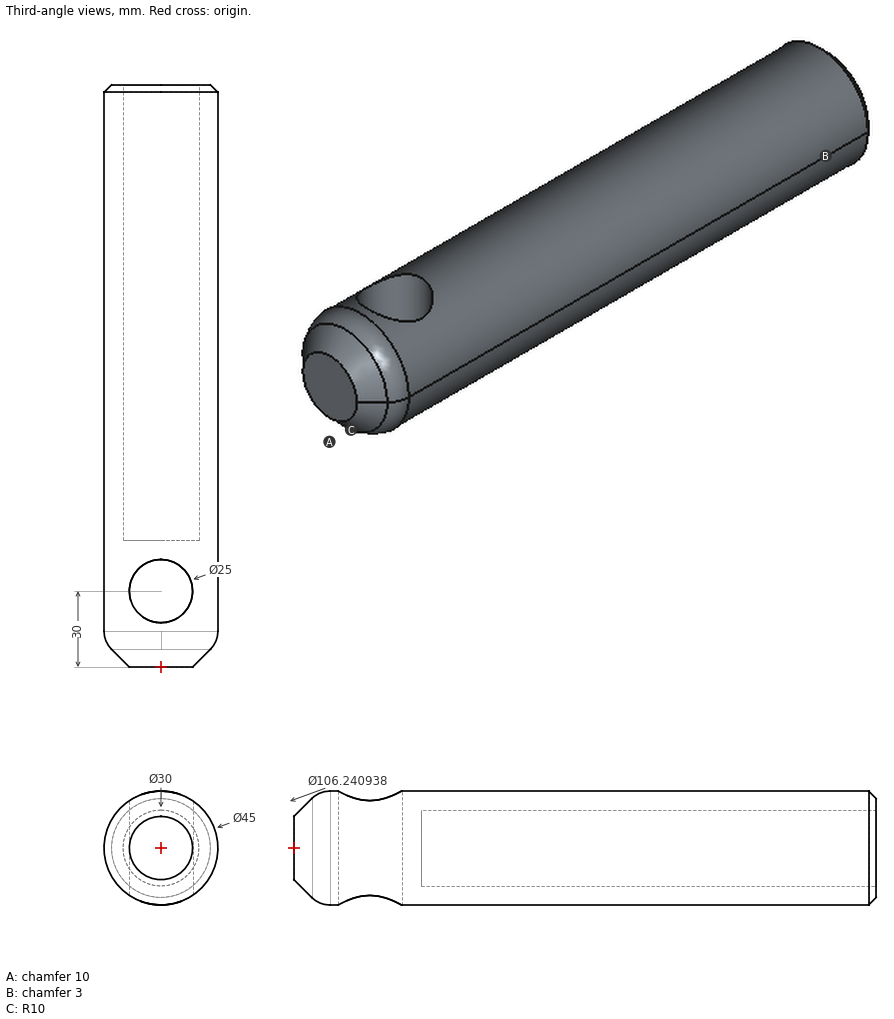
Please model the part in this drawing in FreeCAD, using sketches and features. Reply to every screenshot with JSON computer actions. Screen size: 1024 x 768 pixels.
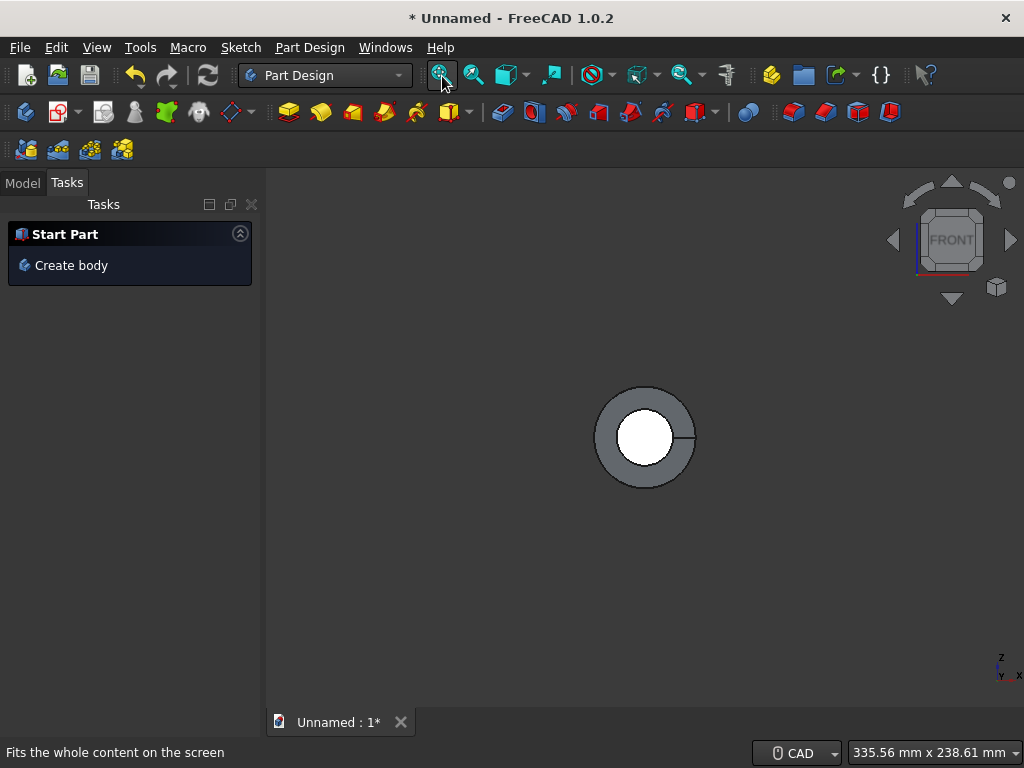
{"action": "key", "text": "3"}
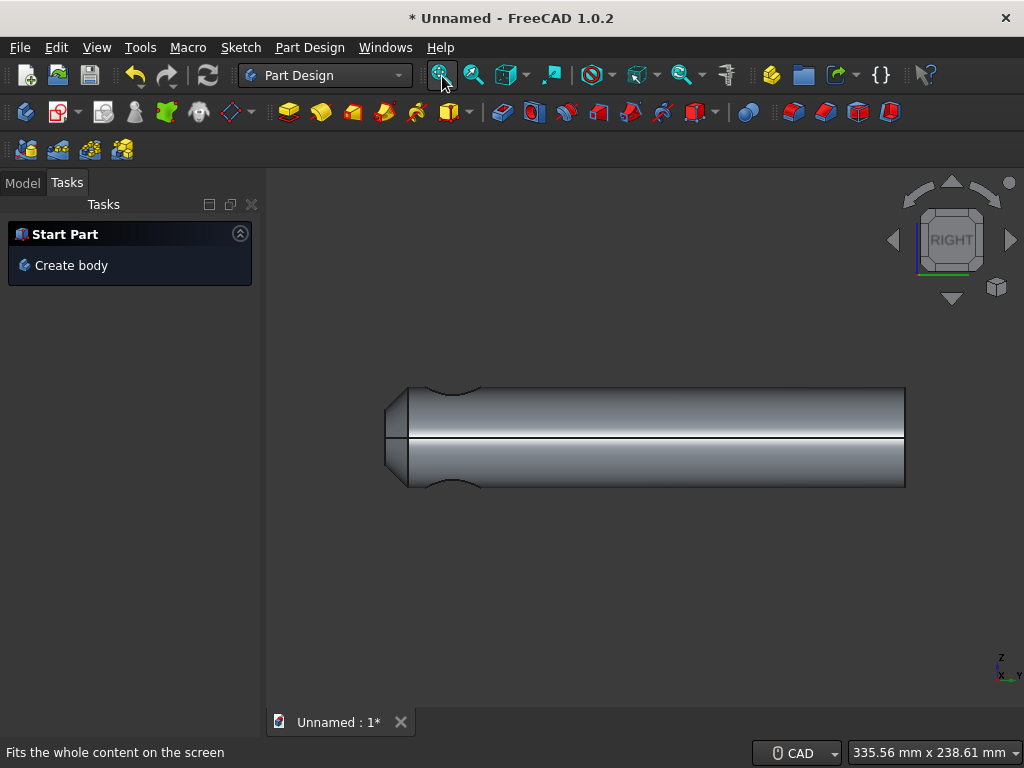
{"action": "left_click", "coordinate": [905, 407]}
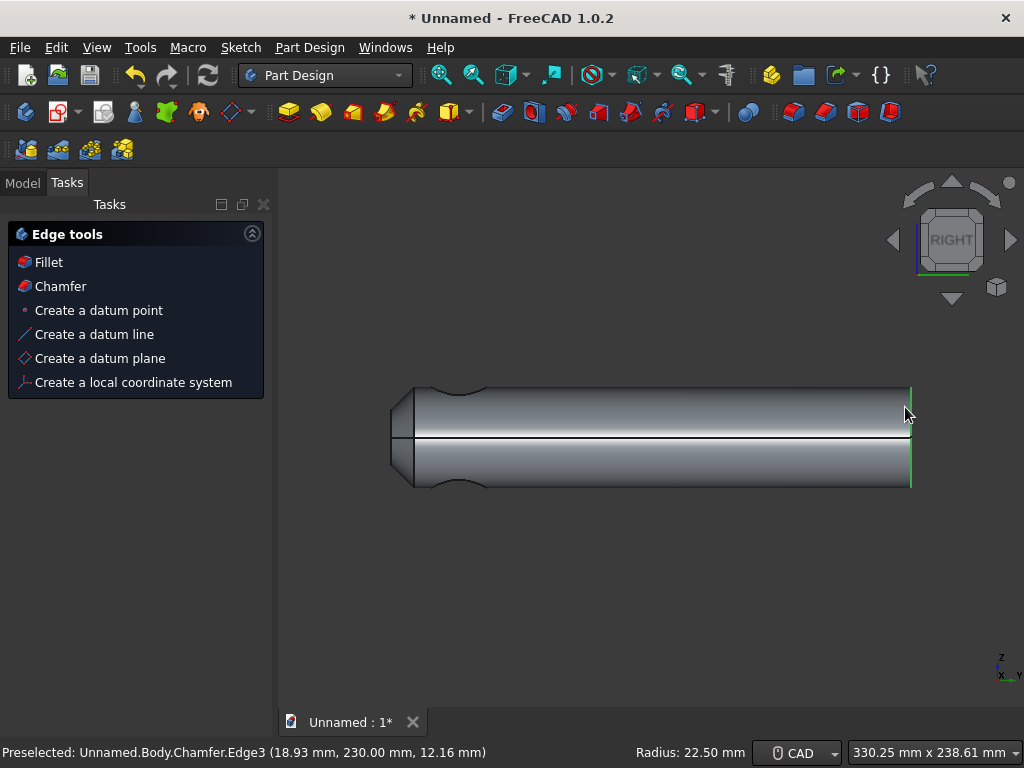
{"action": "left_click", "coordinate": [826, 112]}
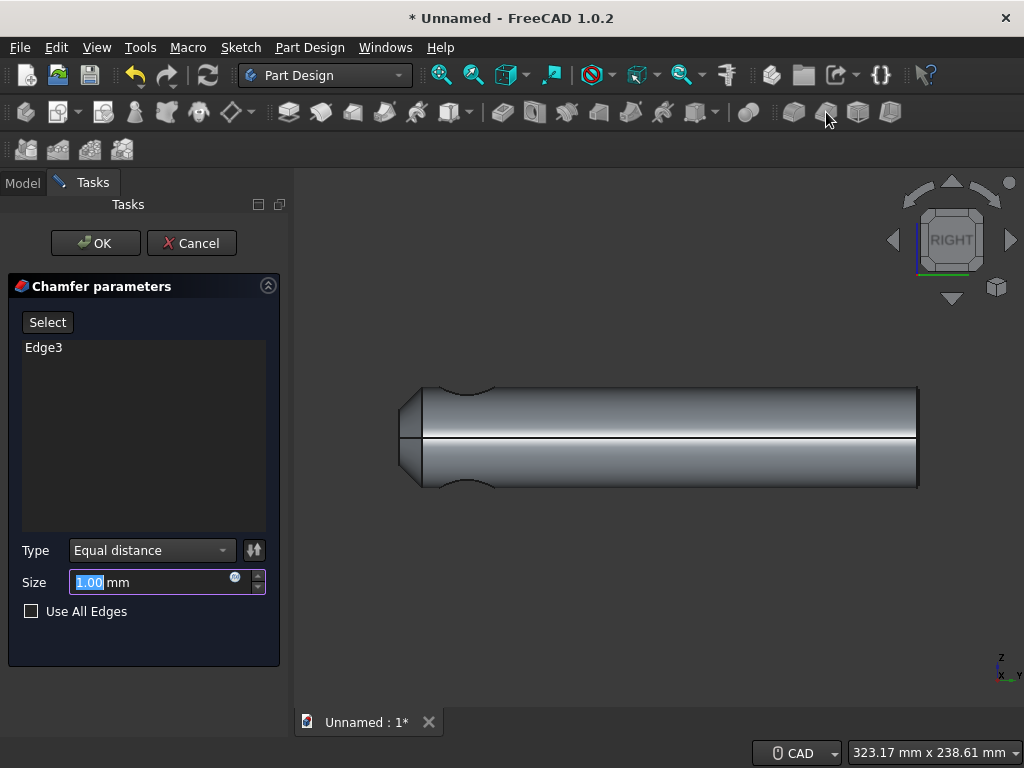
{"action": "type", "text": "3"}
{"action": "key", "text": "Tab"}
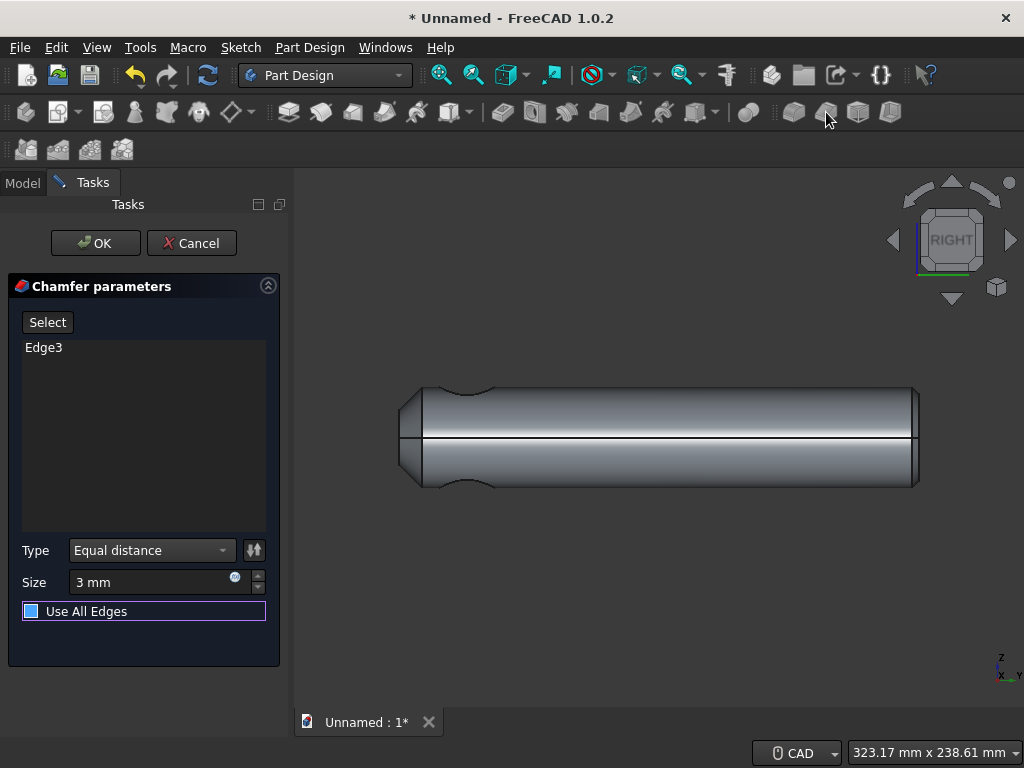
{"action": "left_click", "coordinate": [96, 243]}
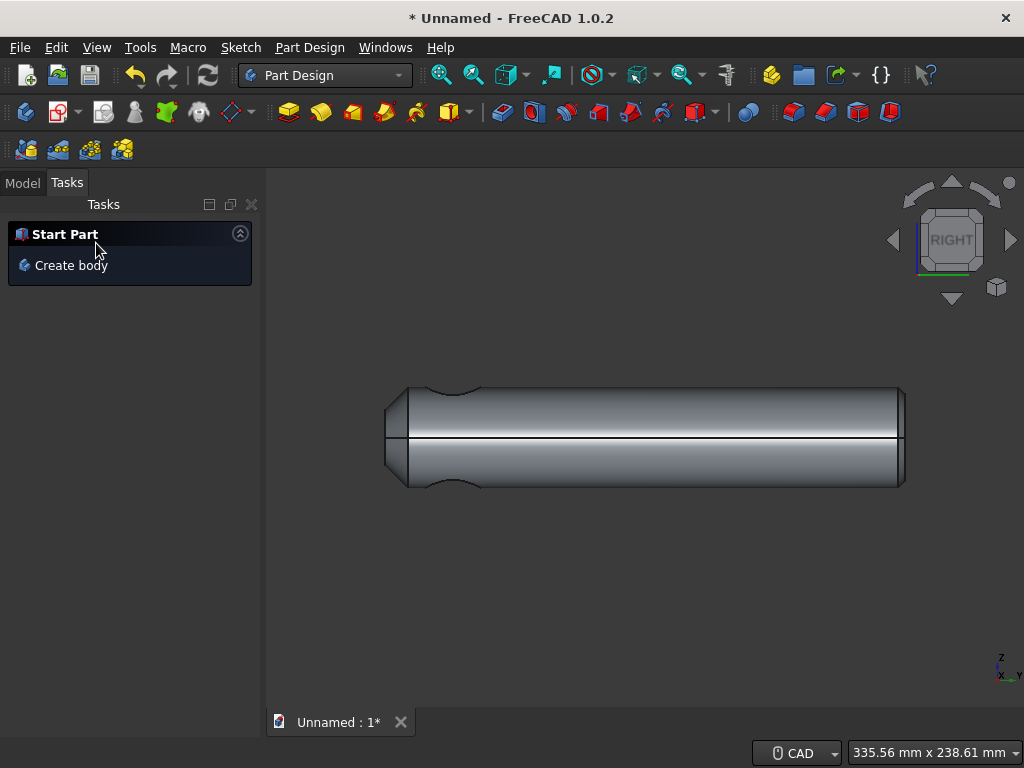
{"action": "left_click", "coordinate": [408, 407]}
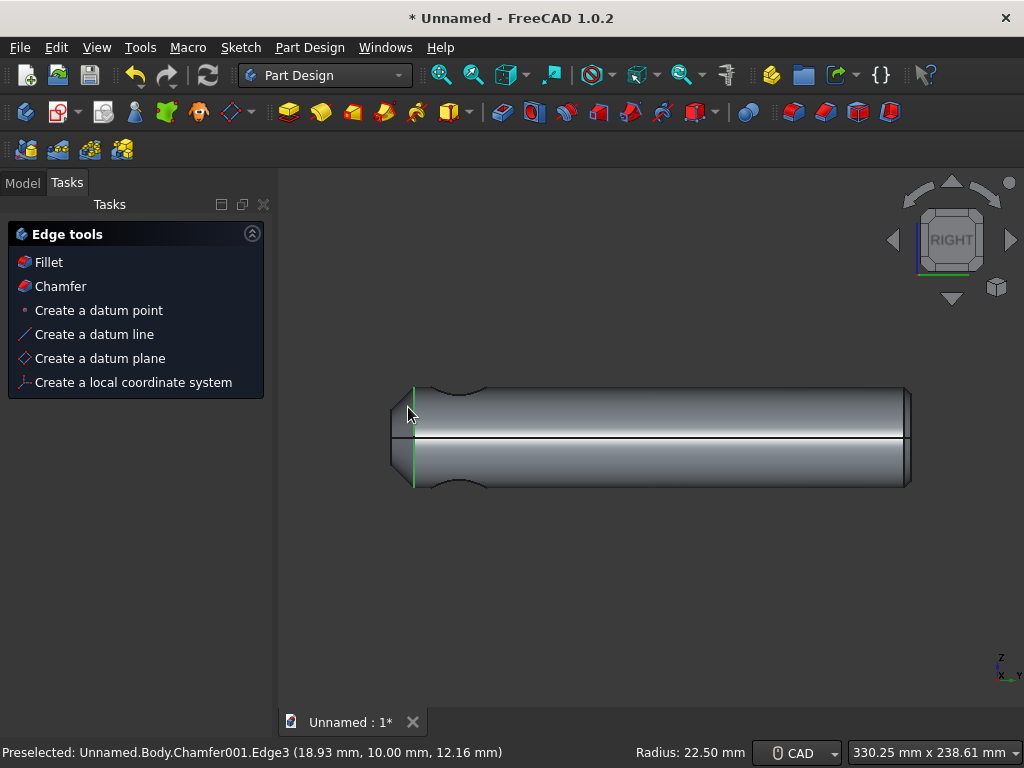
{"action": "left_click", "coordinate": [794, 112]}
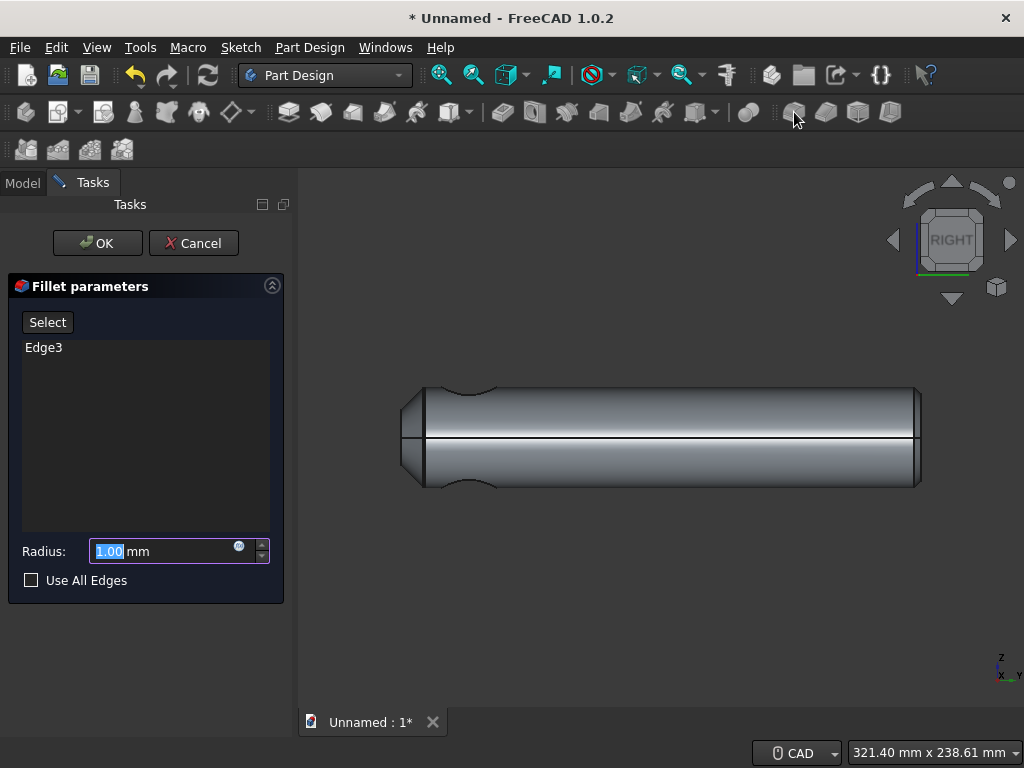
{"action": "type", "text": "10"}
{"action": "key", "text": "Tab"}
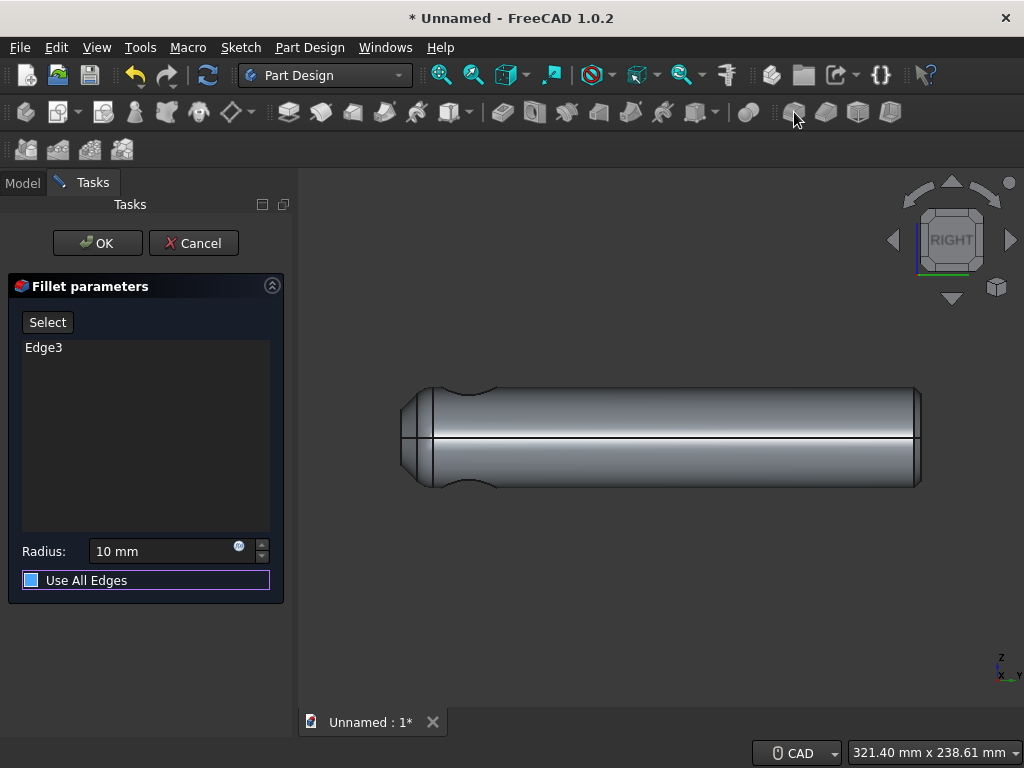
{"action": "left_click", "coordinate": [98, 243]}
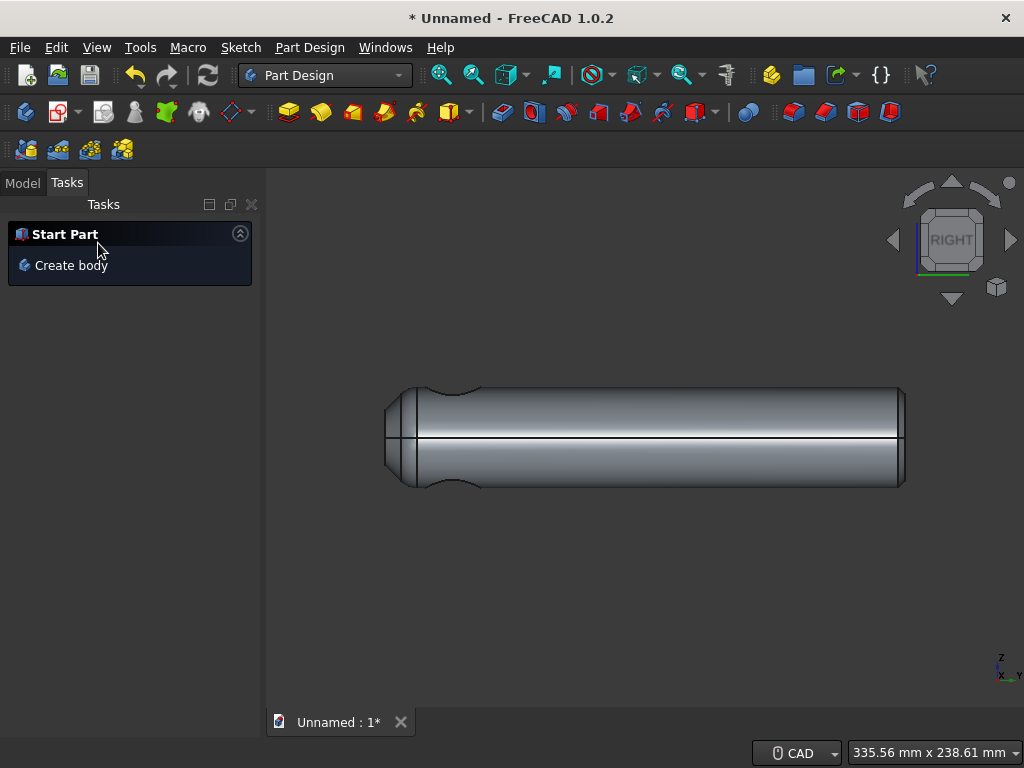
{"action": "key", "text": "0"}